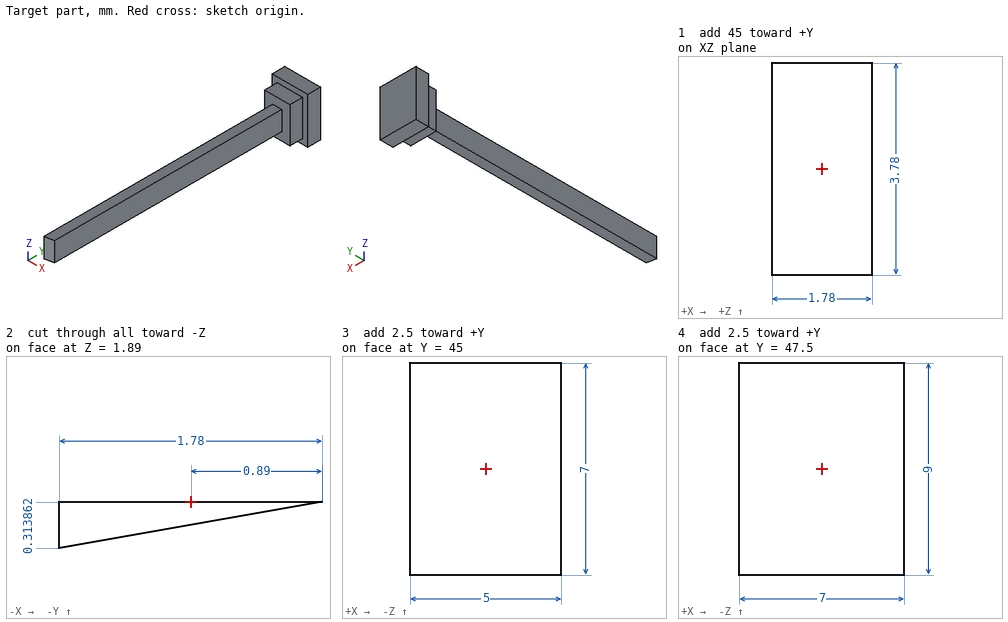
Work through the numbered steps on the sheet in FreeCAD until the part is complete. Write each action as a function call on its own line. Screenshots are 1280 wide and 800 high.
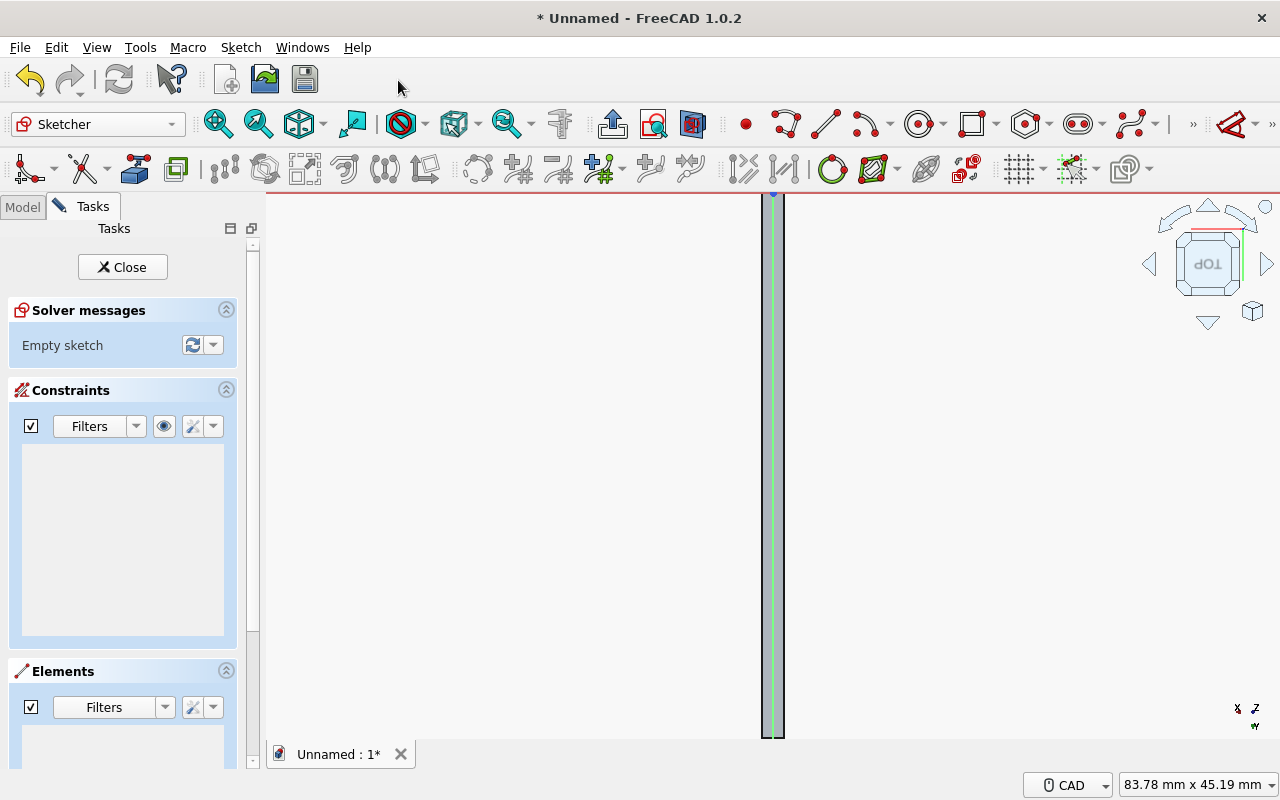
scroll(704, 466, down, 5)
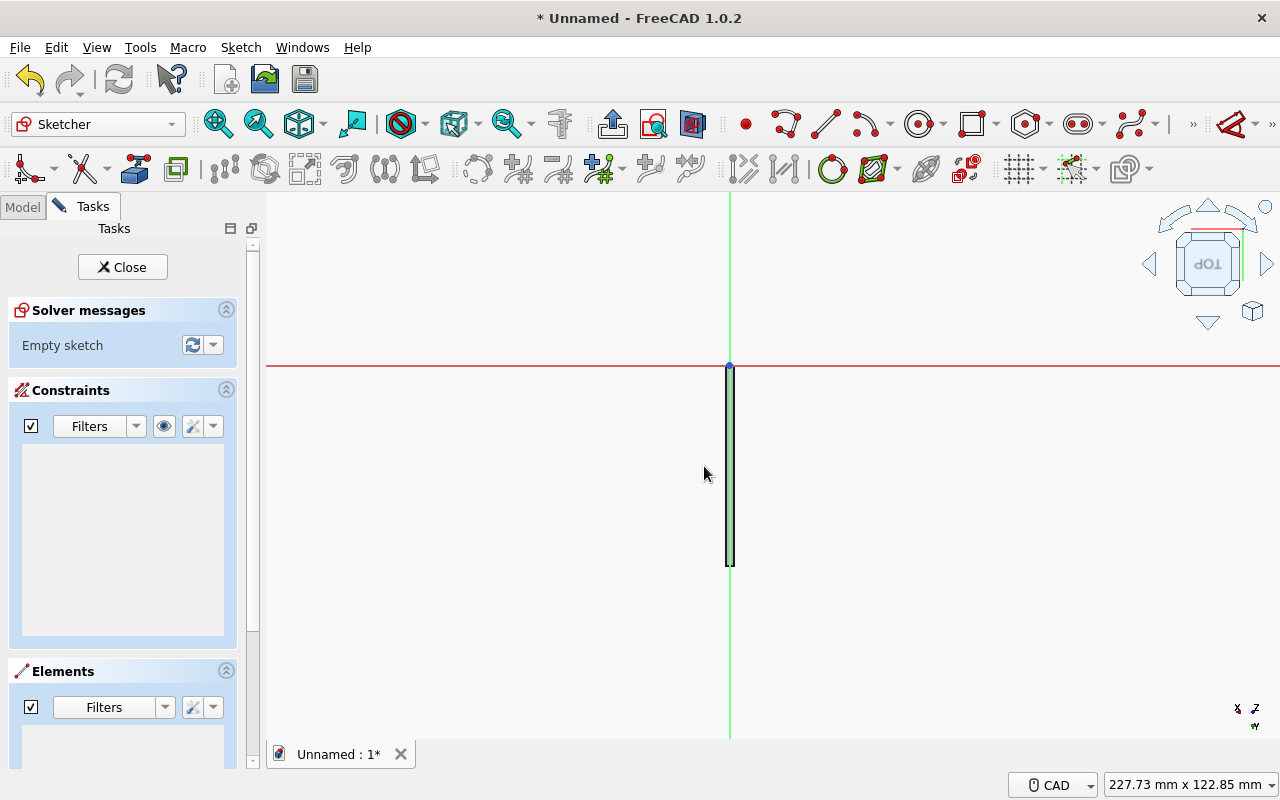
scroll(731, 361, up, 15)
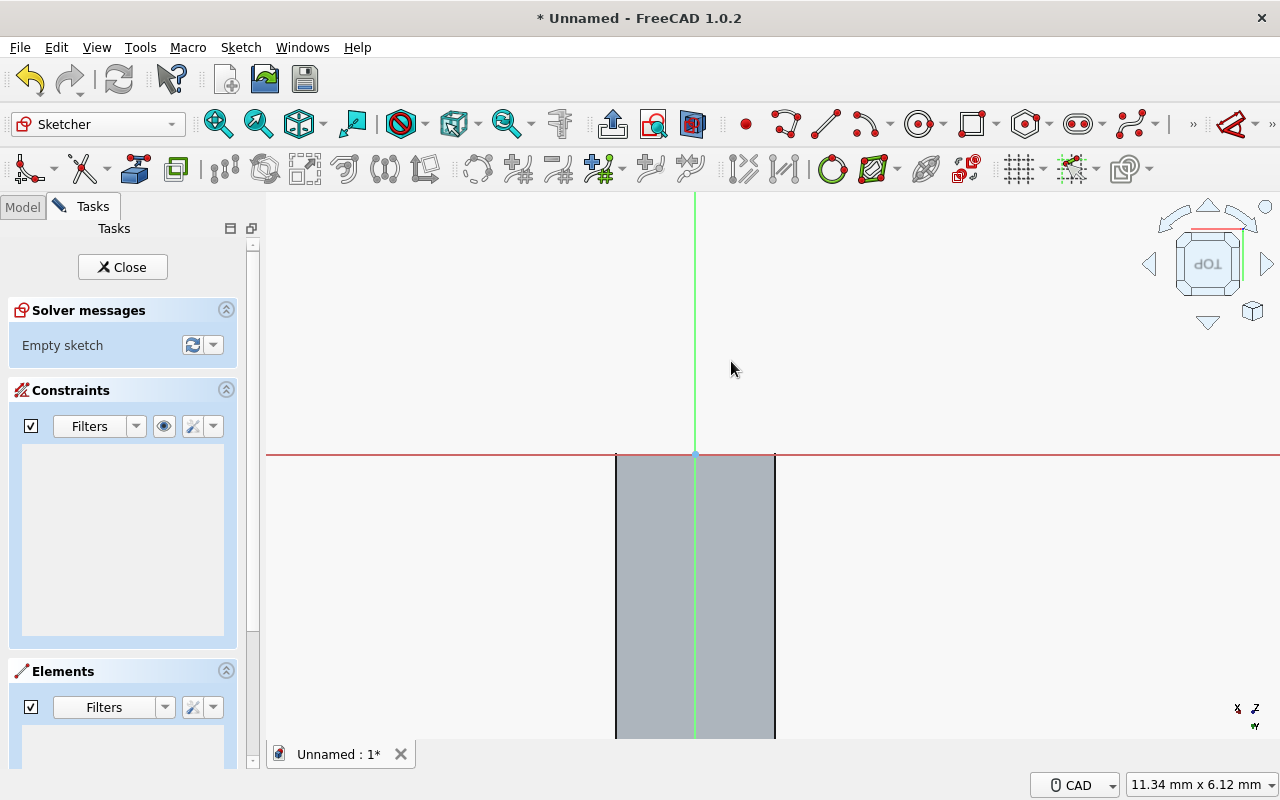
scroll(691, 470, up, 6)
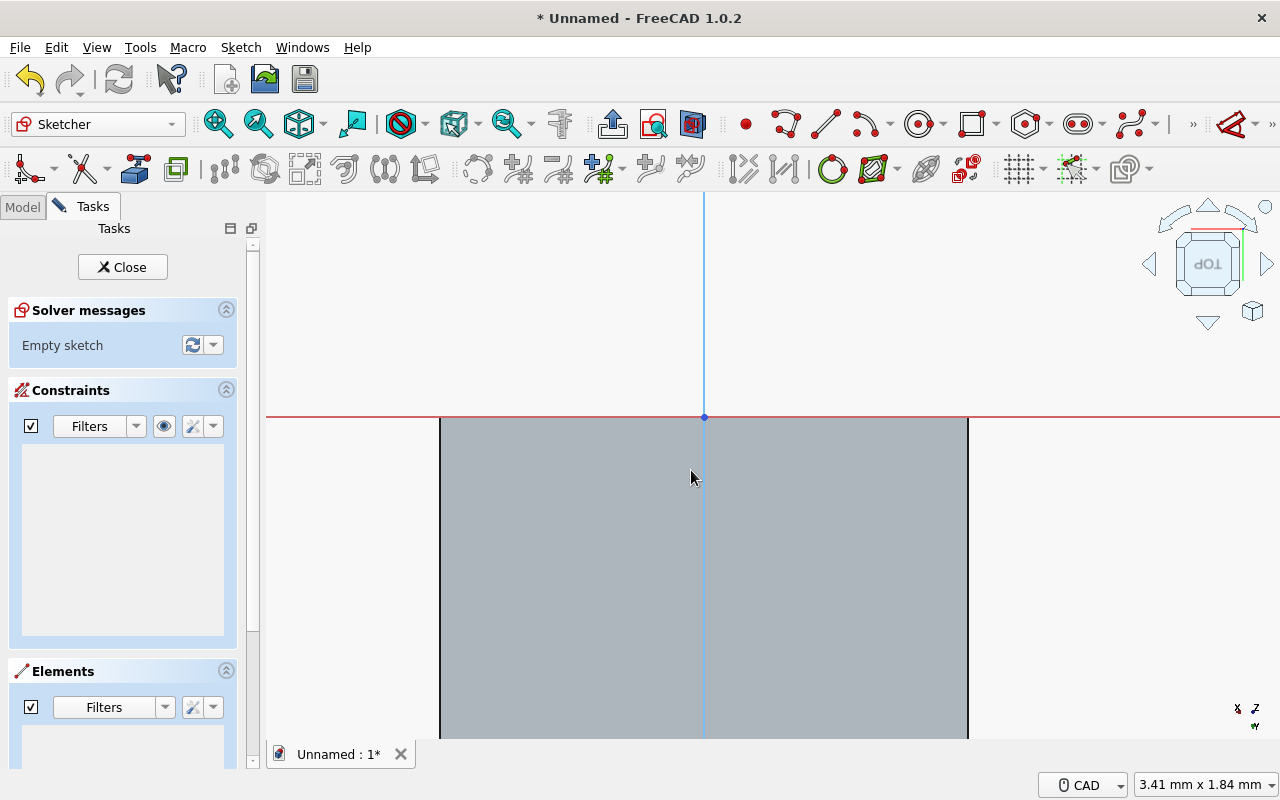
key(g)
key(m)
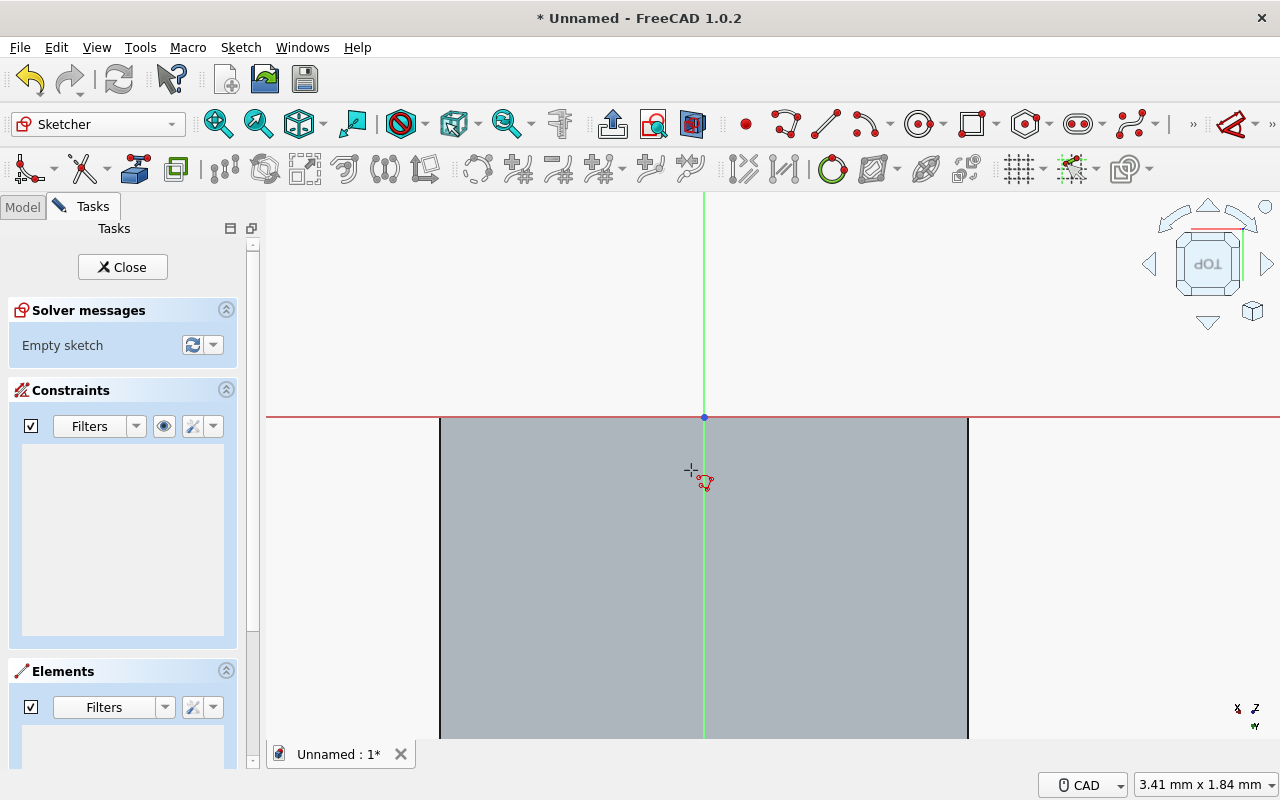
click(968, 417)
click(440, 426)
click(440, 511)
click(968, 417)
key(Escape)
key(Escape)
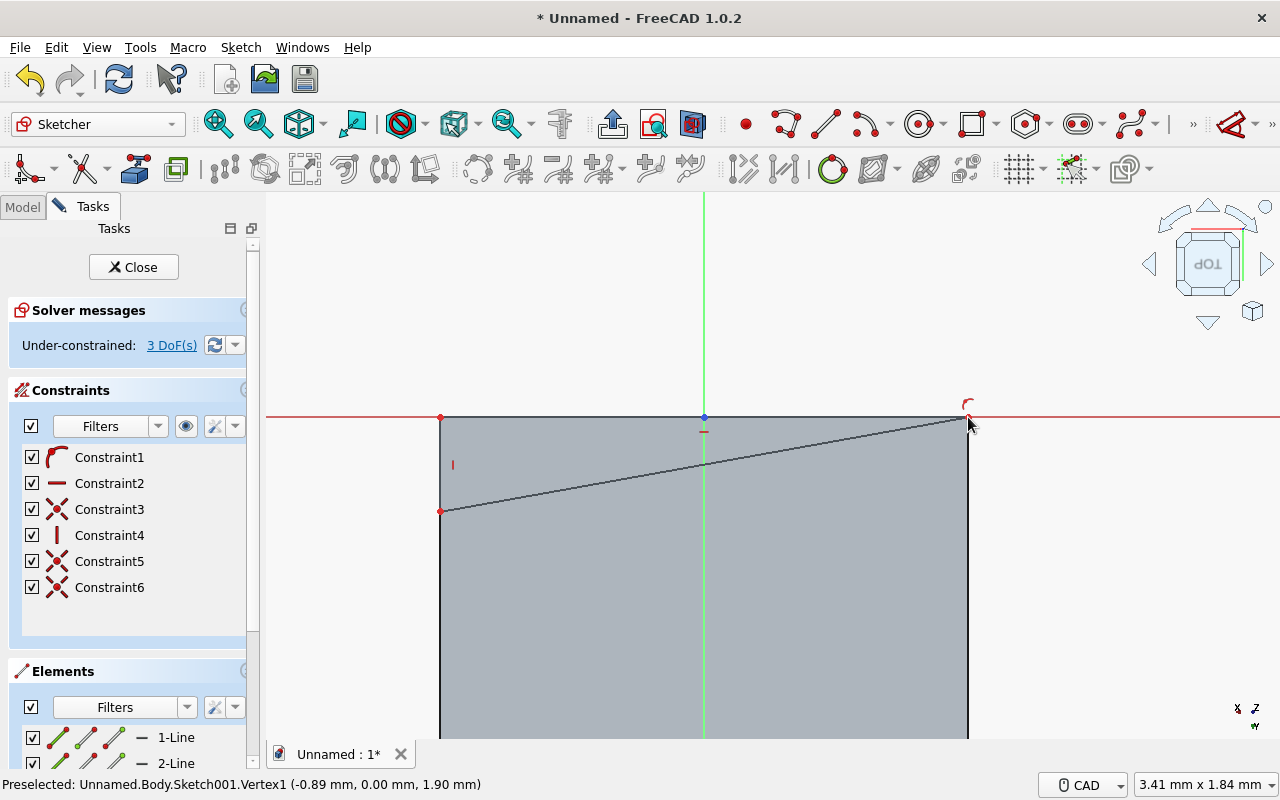
click(1232, 124)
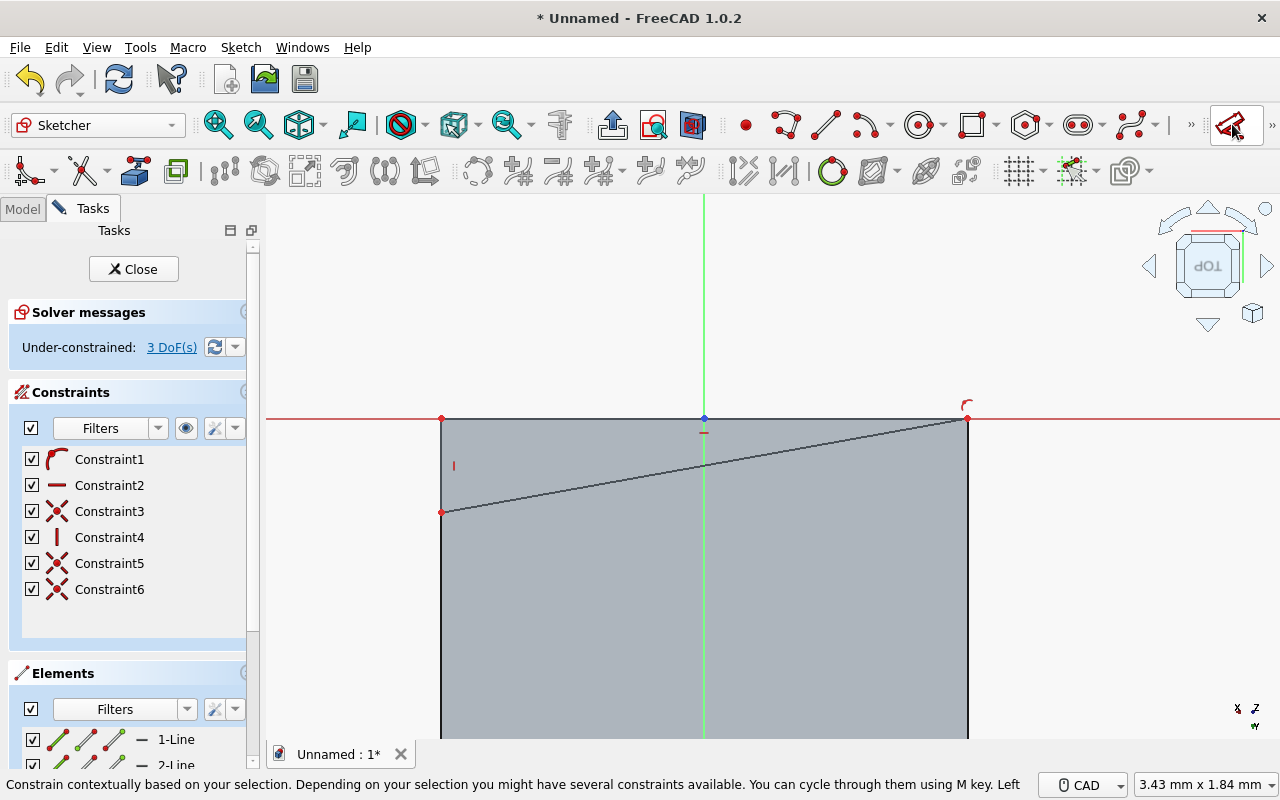
click(809, 419)
click(583, 385)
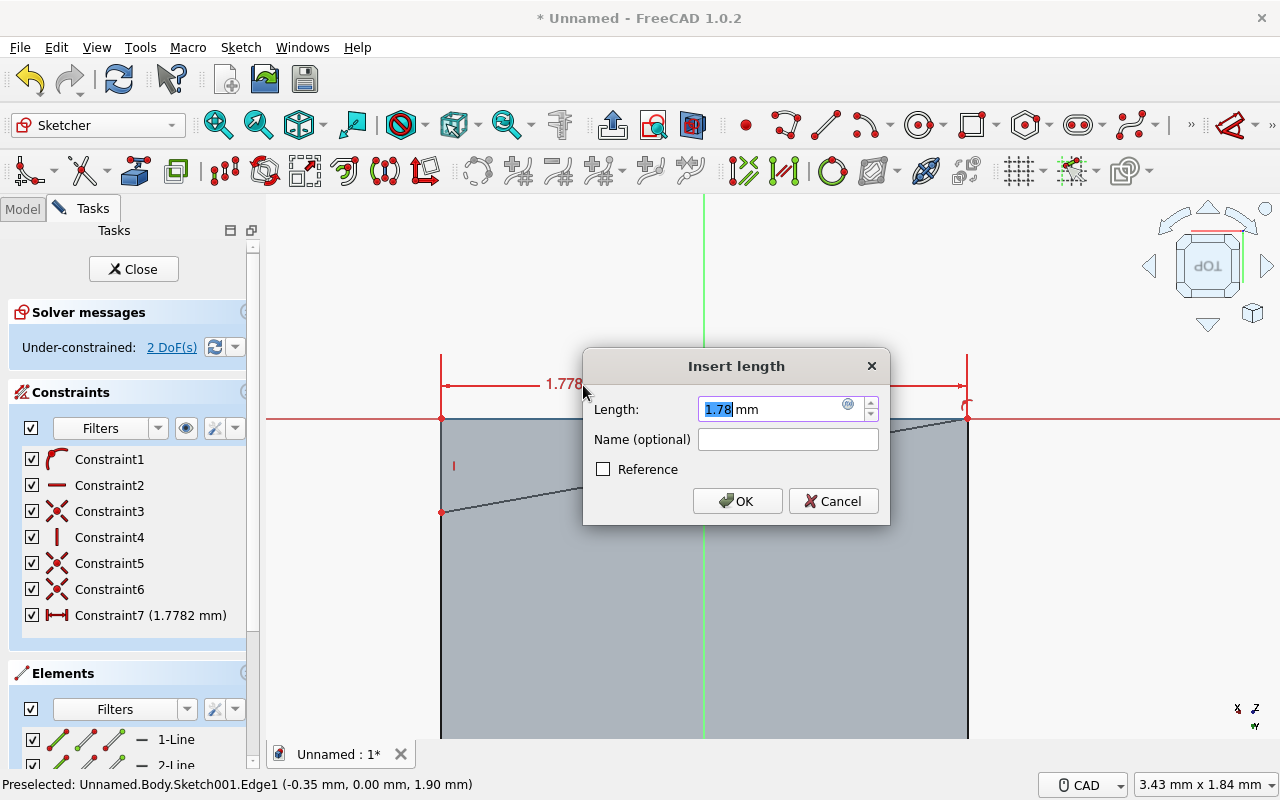
text(1.78)
key(Return)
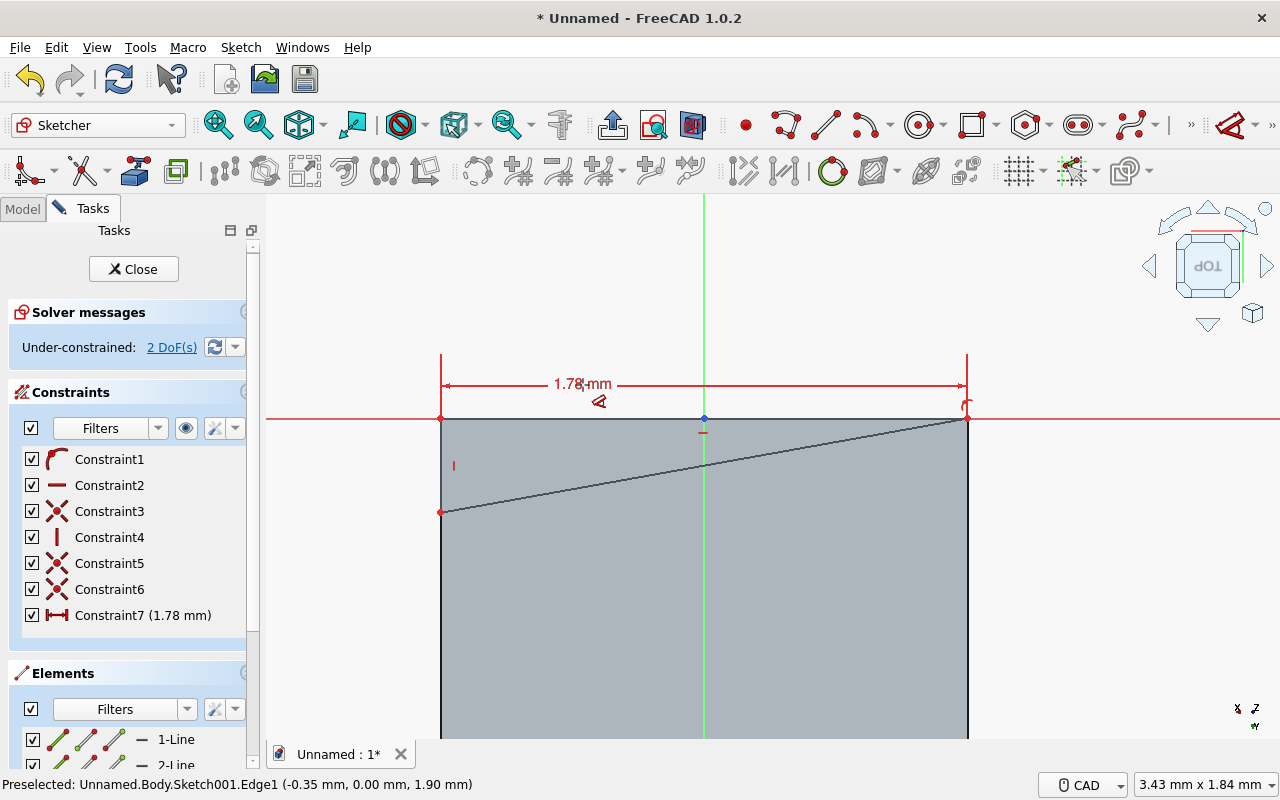
click(967, 419)
click(836, 385)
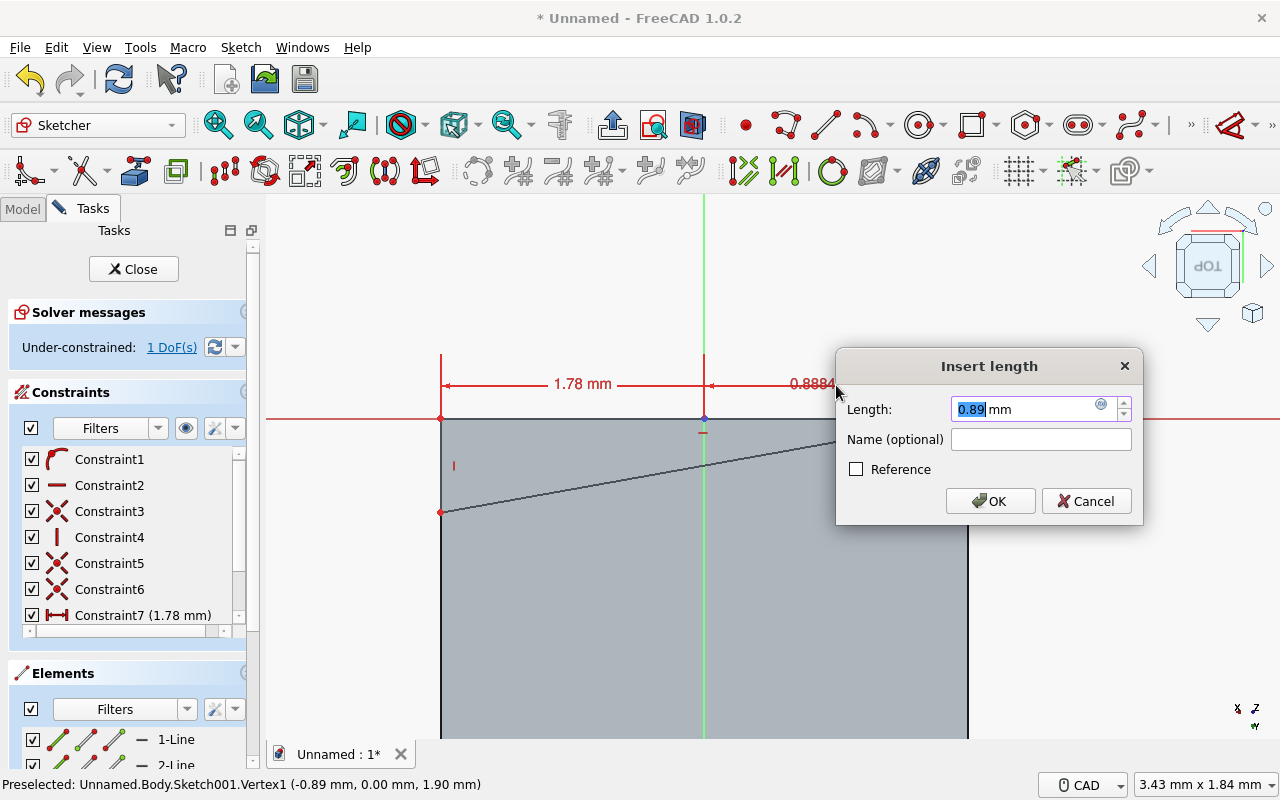
text(0.89)
key(Return)